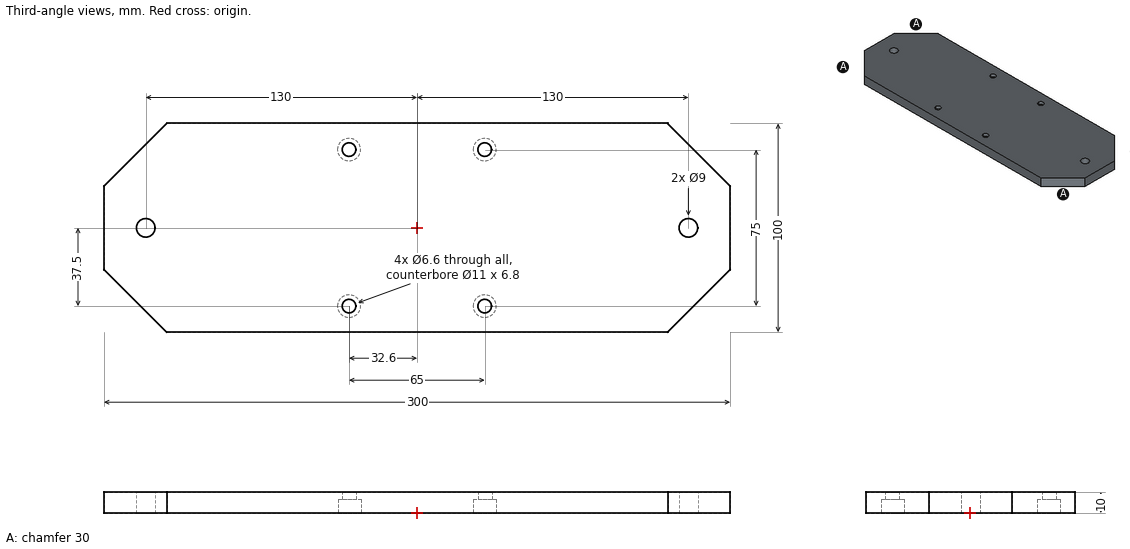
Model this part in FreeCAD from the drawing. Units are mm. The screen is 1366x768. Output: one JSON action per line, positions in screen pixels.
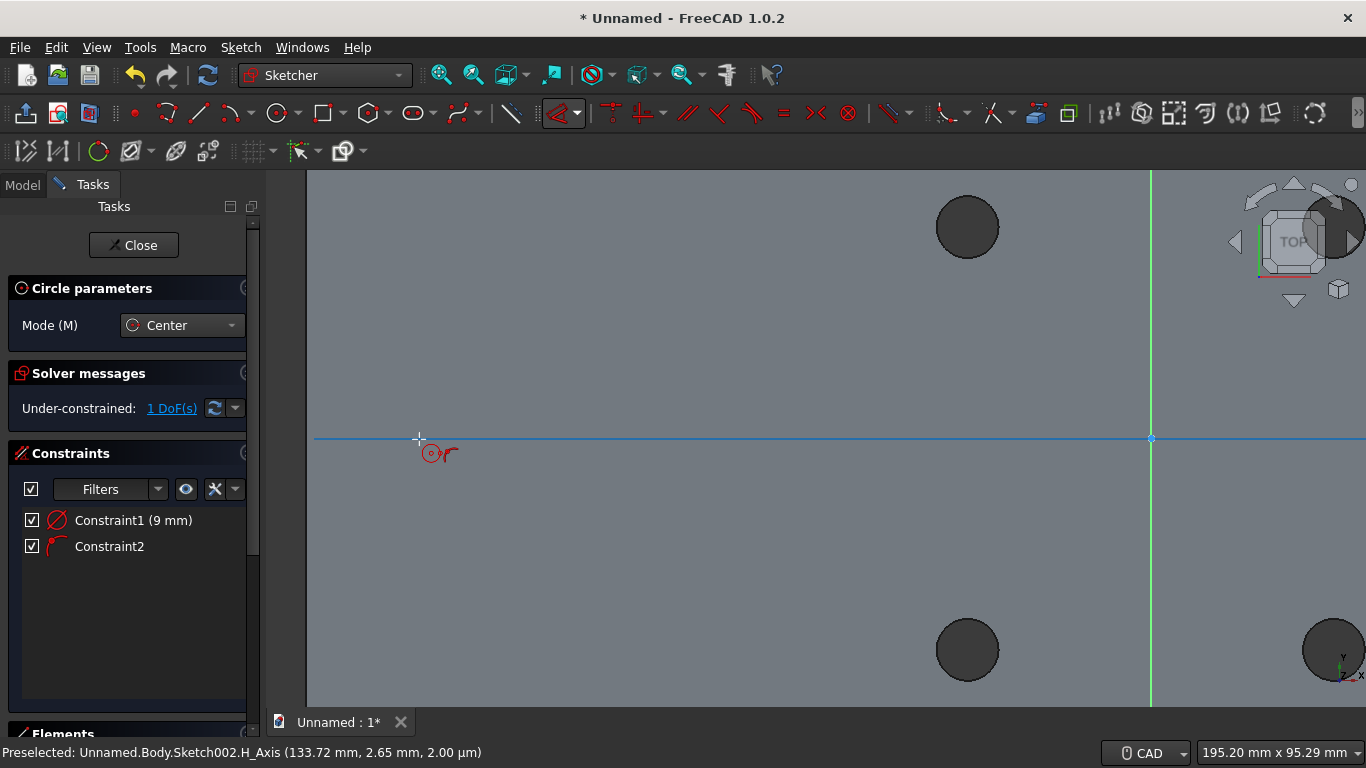
{"action": "left_click", "coordinate": [419, 438]}
{"action": "mouse_move", "coordinate": [437, 421]}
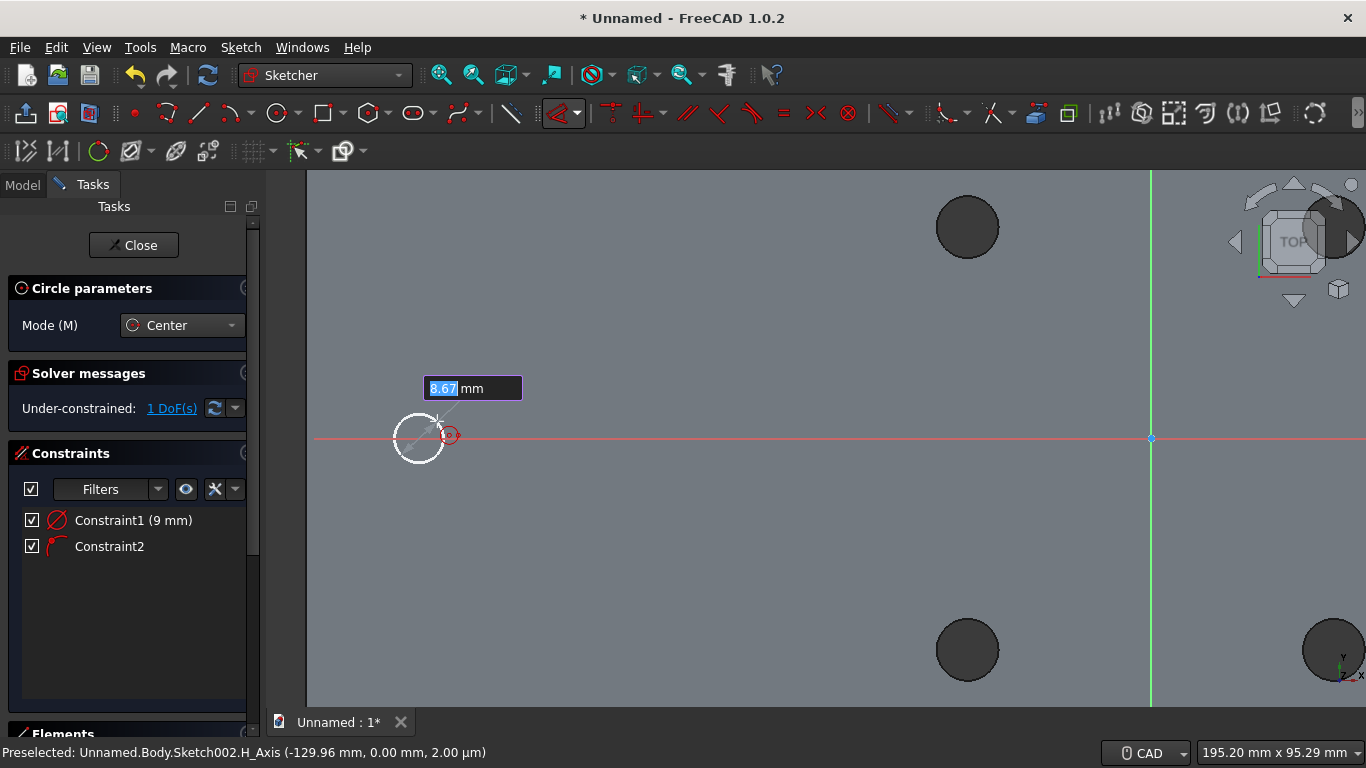
{"action": "type", "text": "9"}
{"action": "key", "text": "Return"}
{"action": "key", "text": "Escape"}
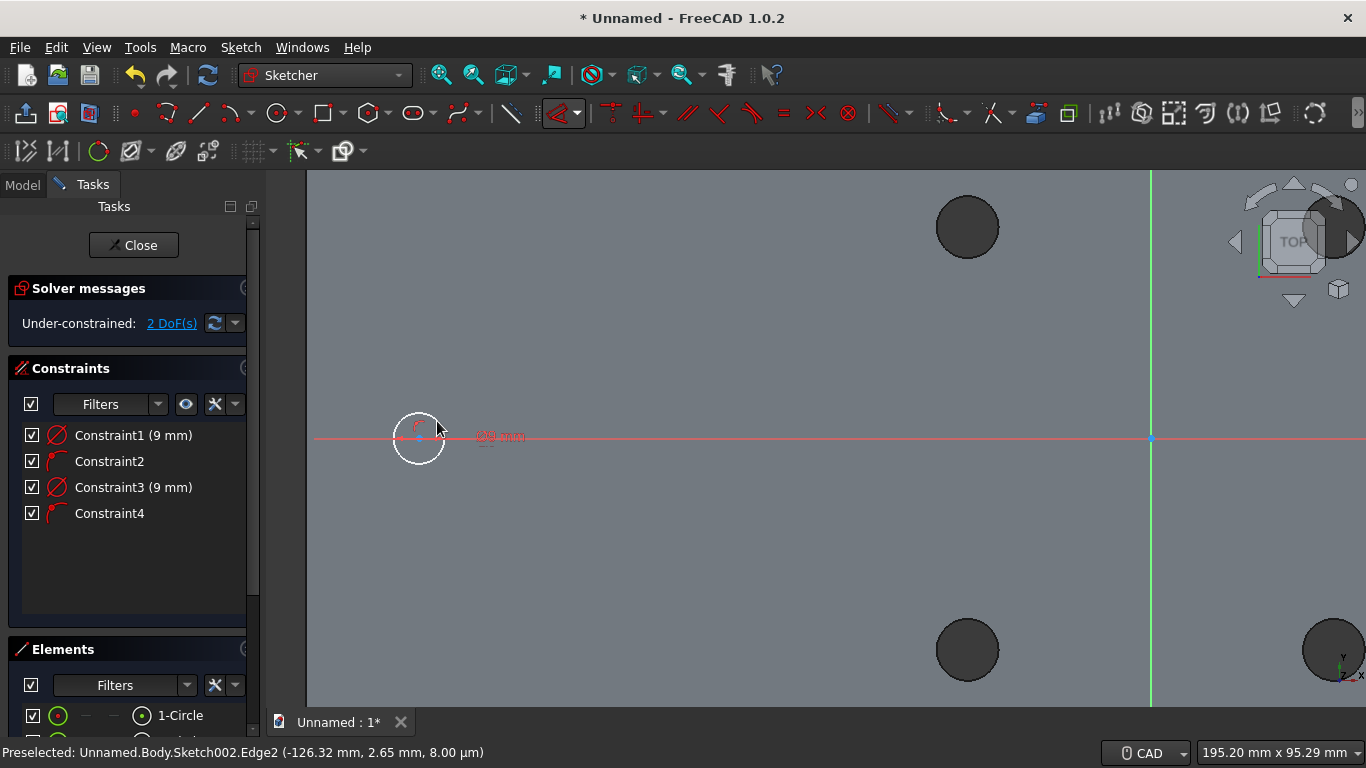
{"action": "scroll", "coordinate": [418, 439], "scroll_direction": "down", "scroll_amount": 4}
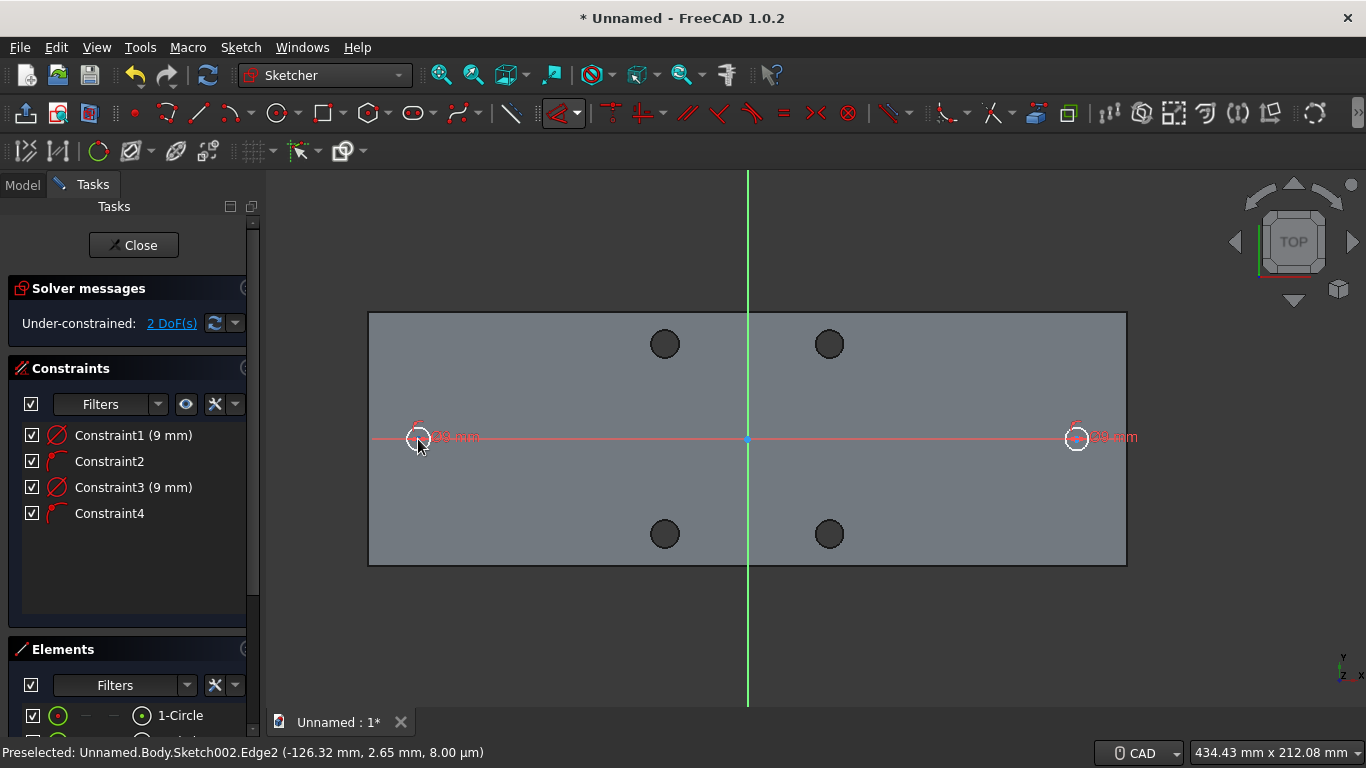
{"action": "left_click", "coordinate": [1077, 439]}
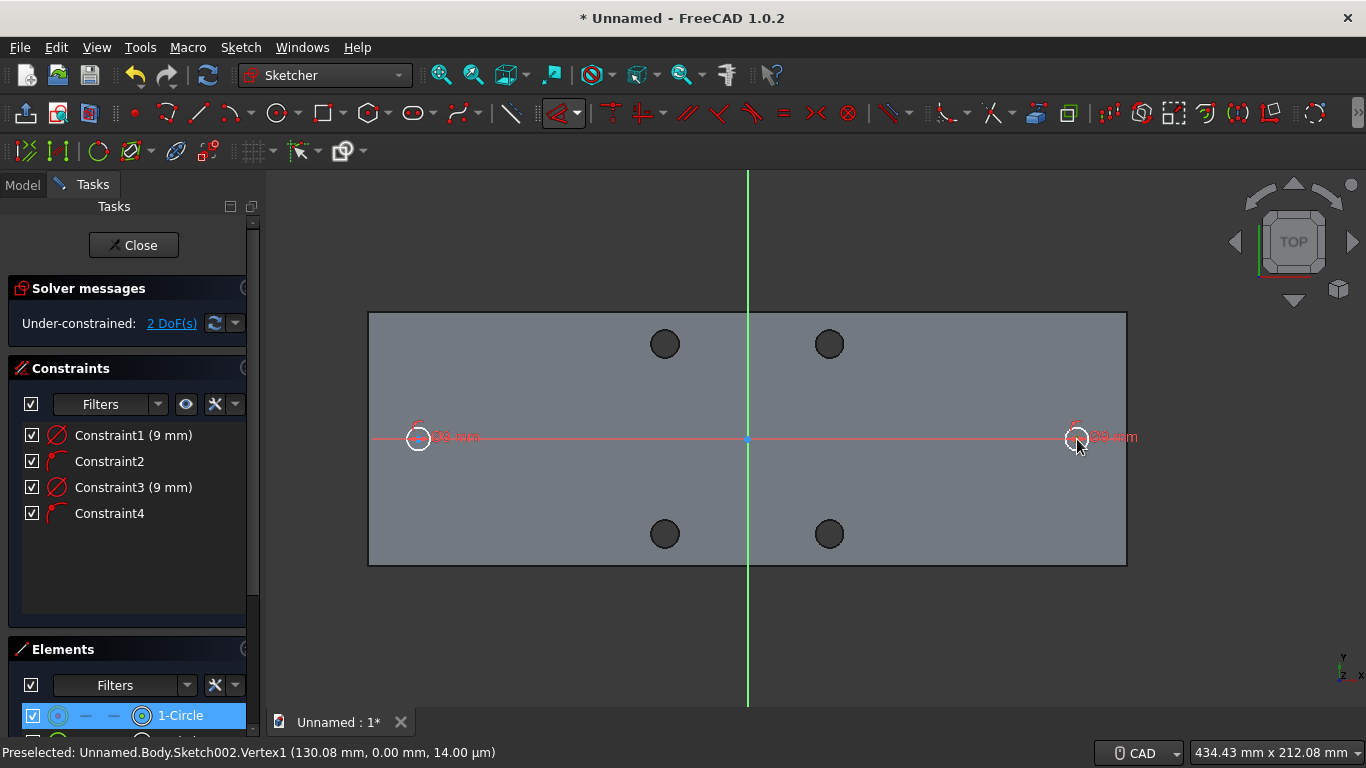
{"action": "key", "text": "l"}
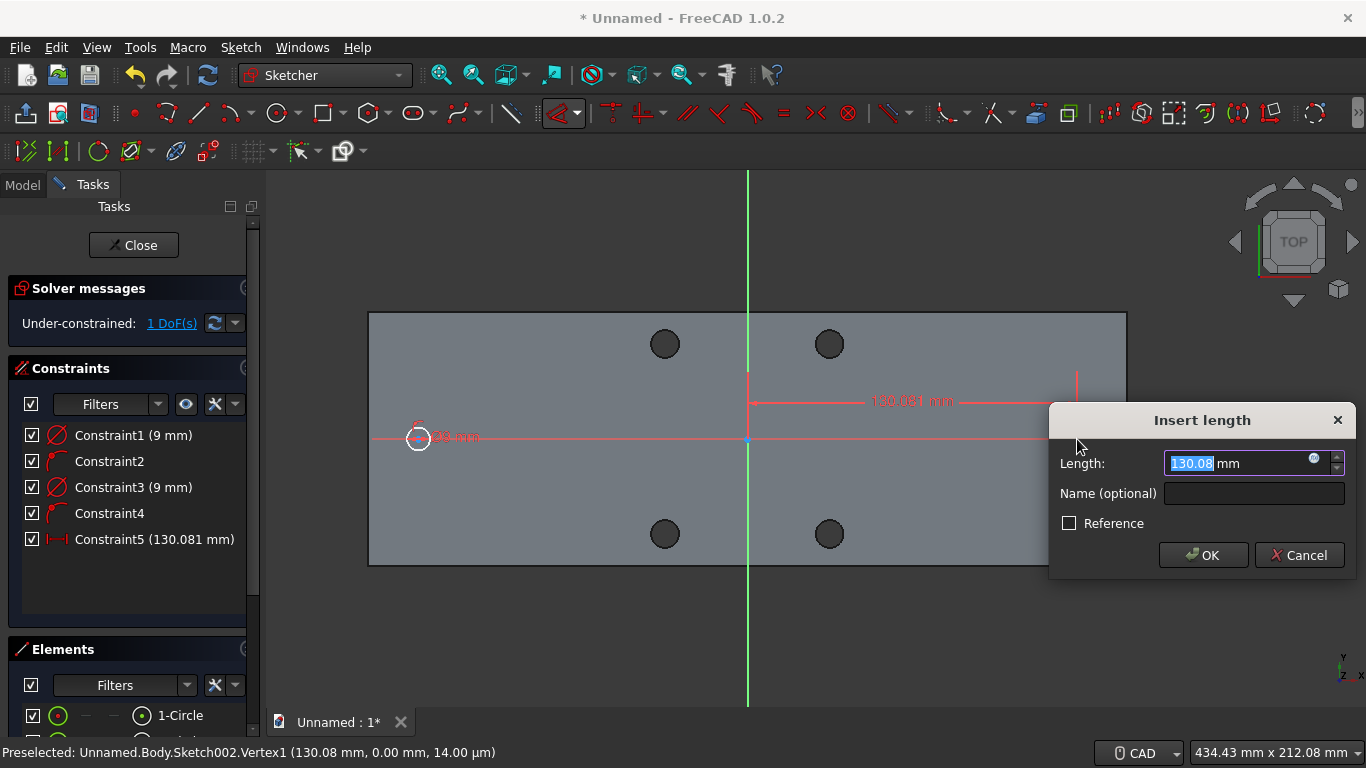
{"action": "type", "text": "130"}
{"action": "key", "text": "Return"}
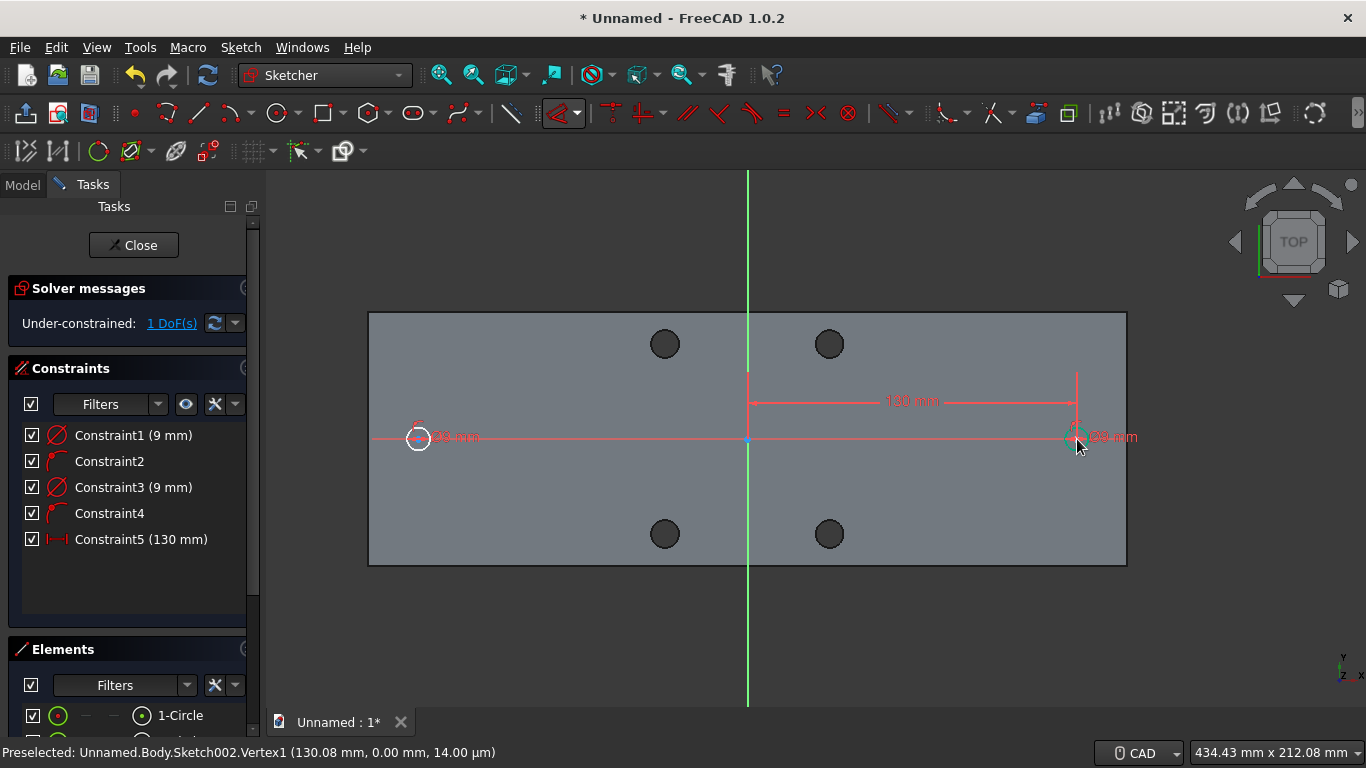
{"action": "left_click", "coordinate": [419, 439]}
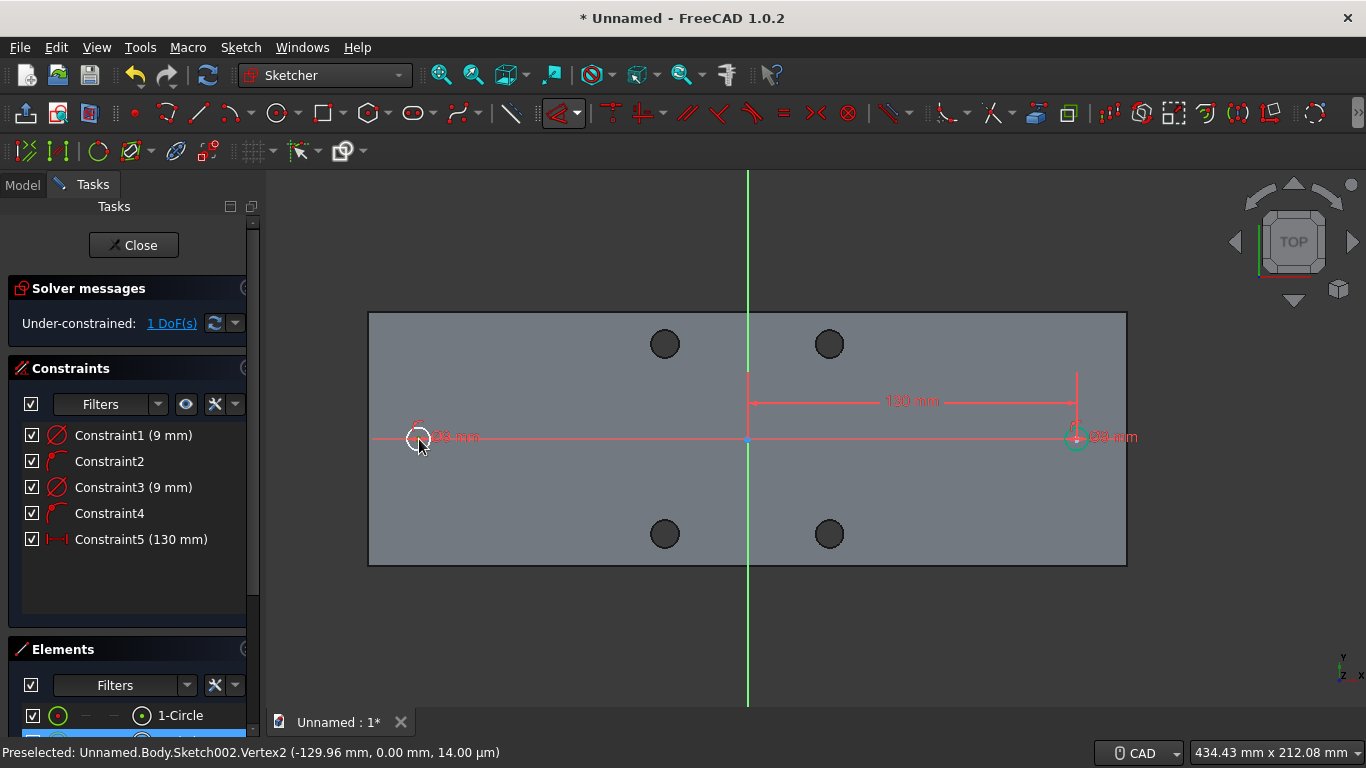
{"action": "left_click", "coordinate": [580, 114]}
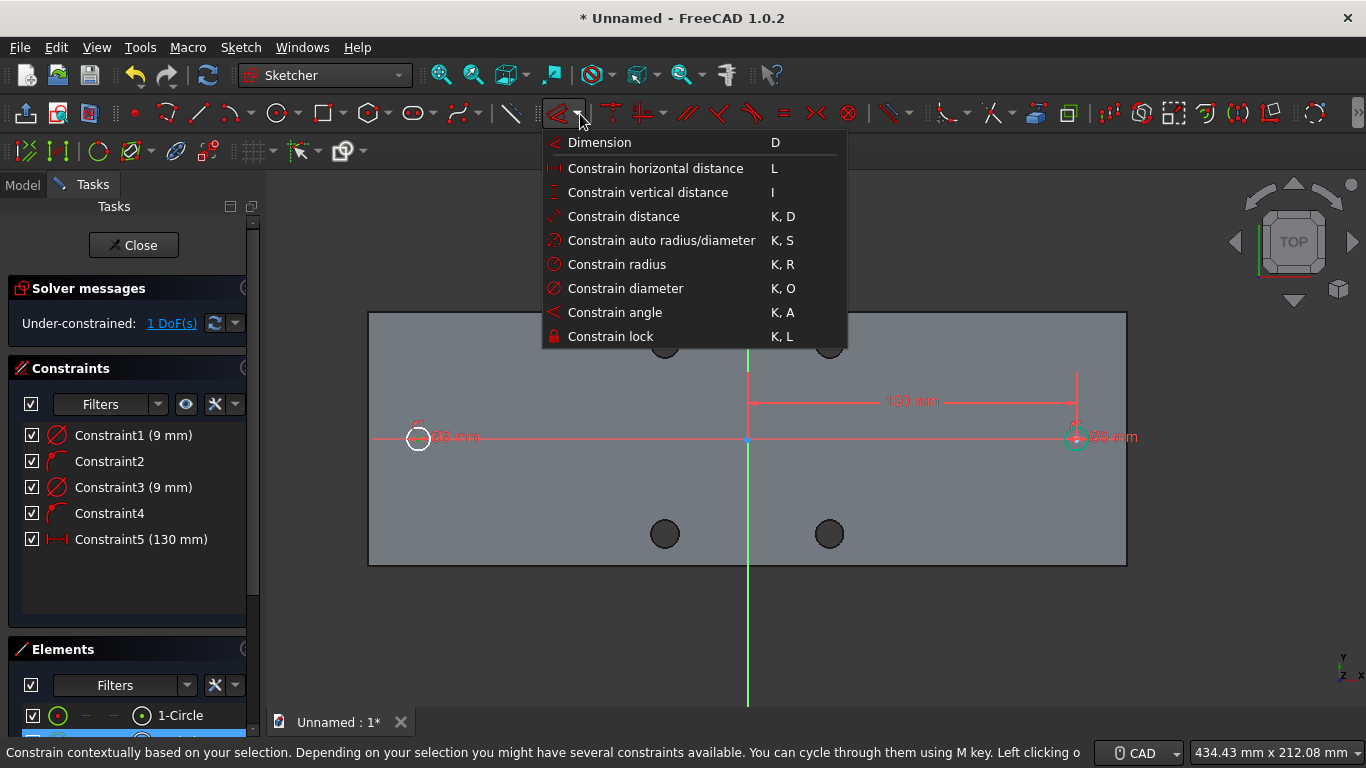
{"action": "left_click", "coordinate": [695, 168]}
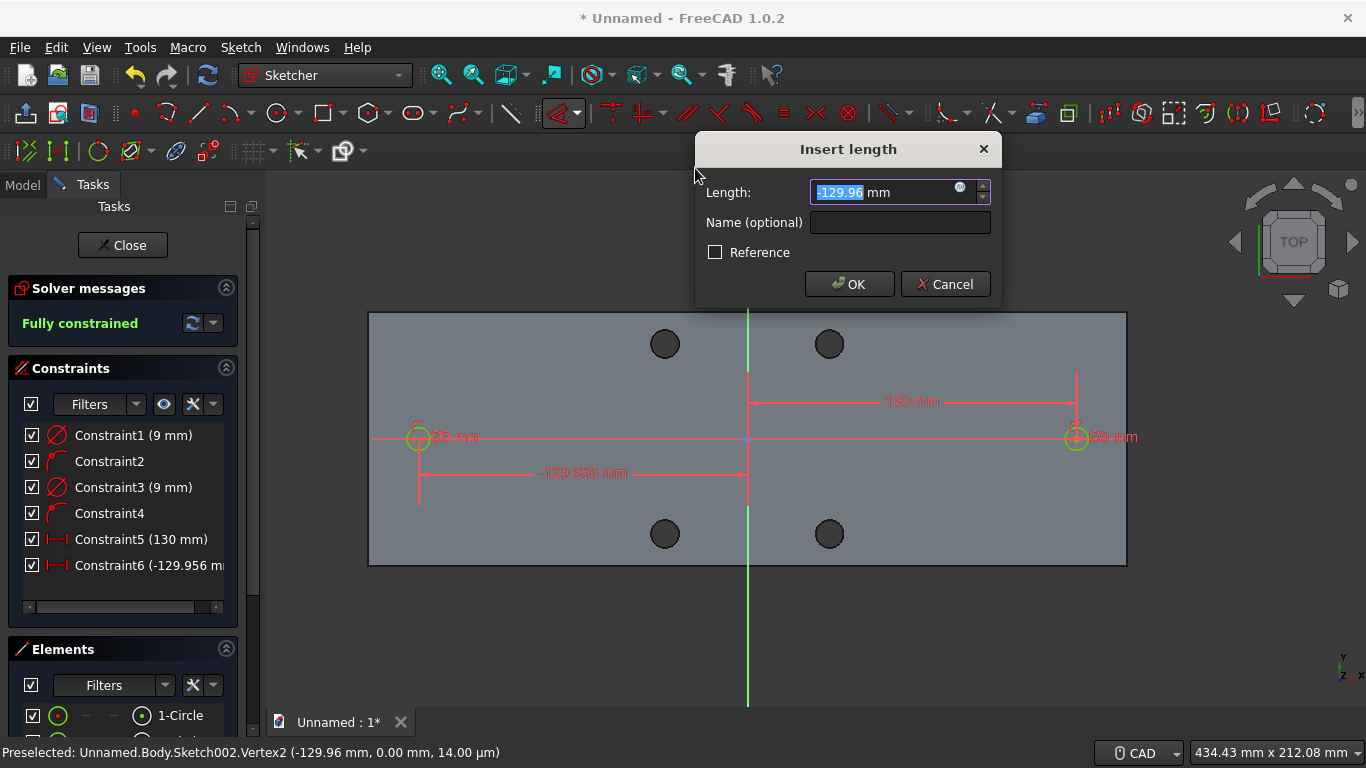
{"action": "type", "text": "-130"}
{"action": "key", "text": "Return"}